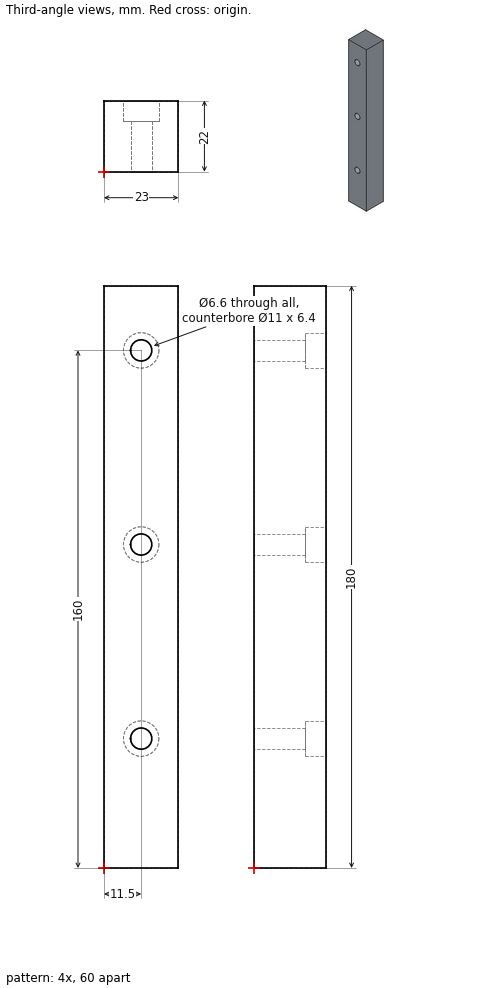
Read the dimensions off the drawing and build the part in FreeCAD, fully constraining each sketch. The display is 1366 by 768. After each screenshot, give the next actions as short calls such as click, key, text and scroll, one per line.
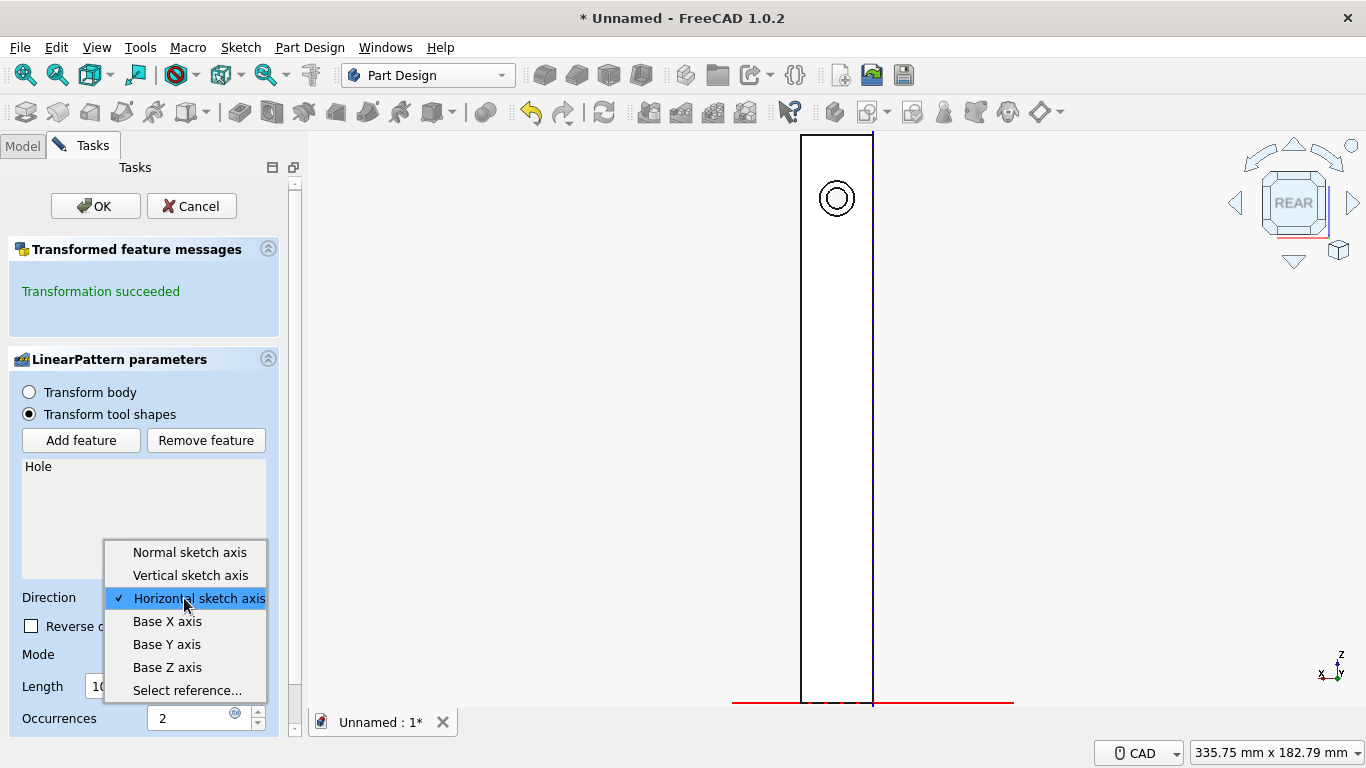
click(184, 668)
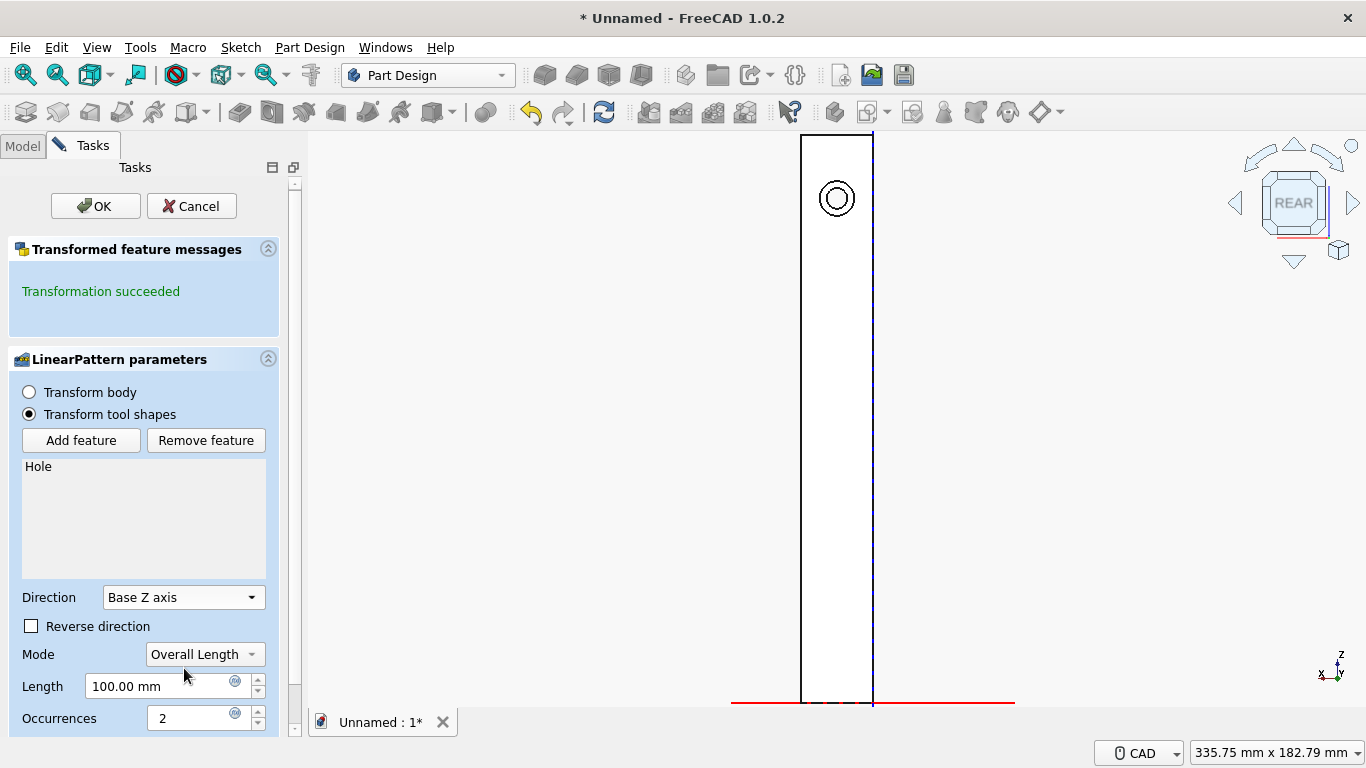
click(206, 654)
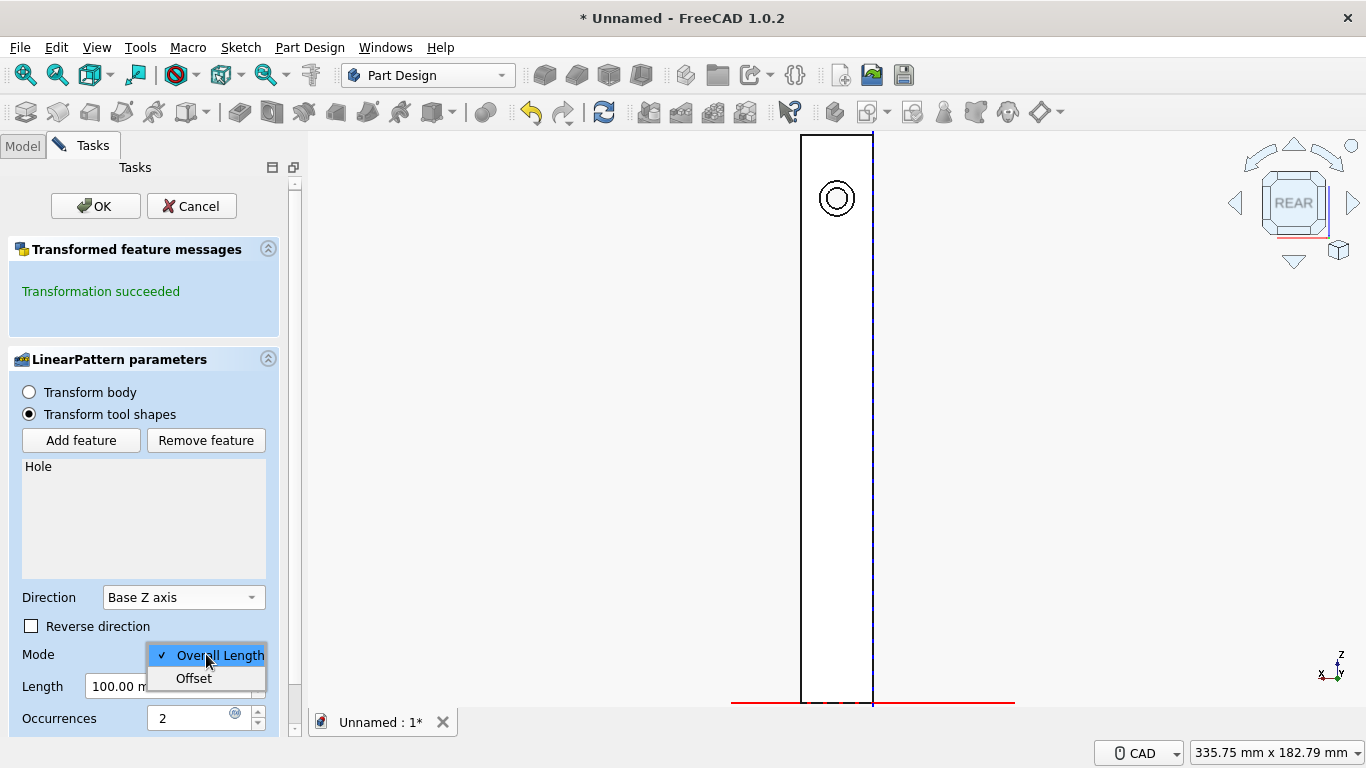
click(206, 678)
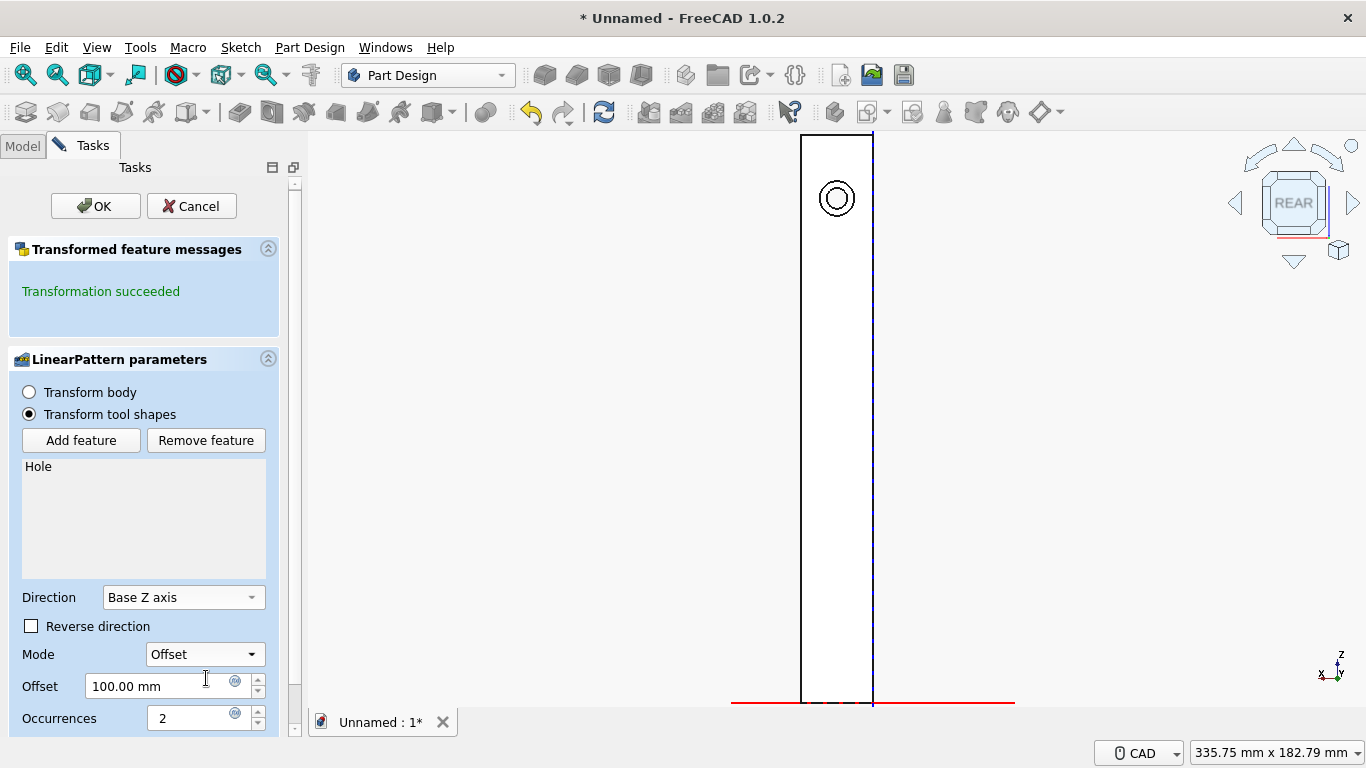
triple_click(168, 686)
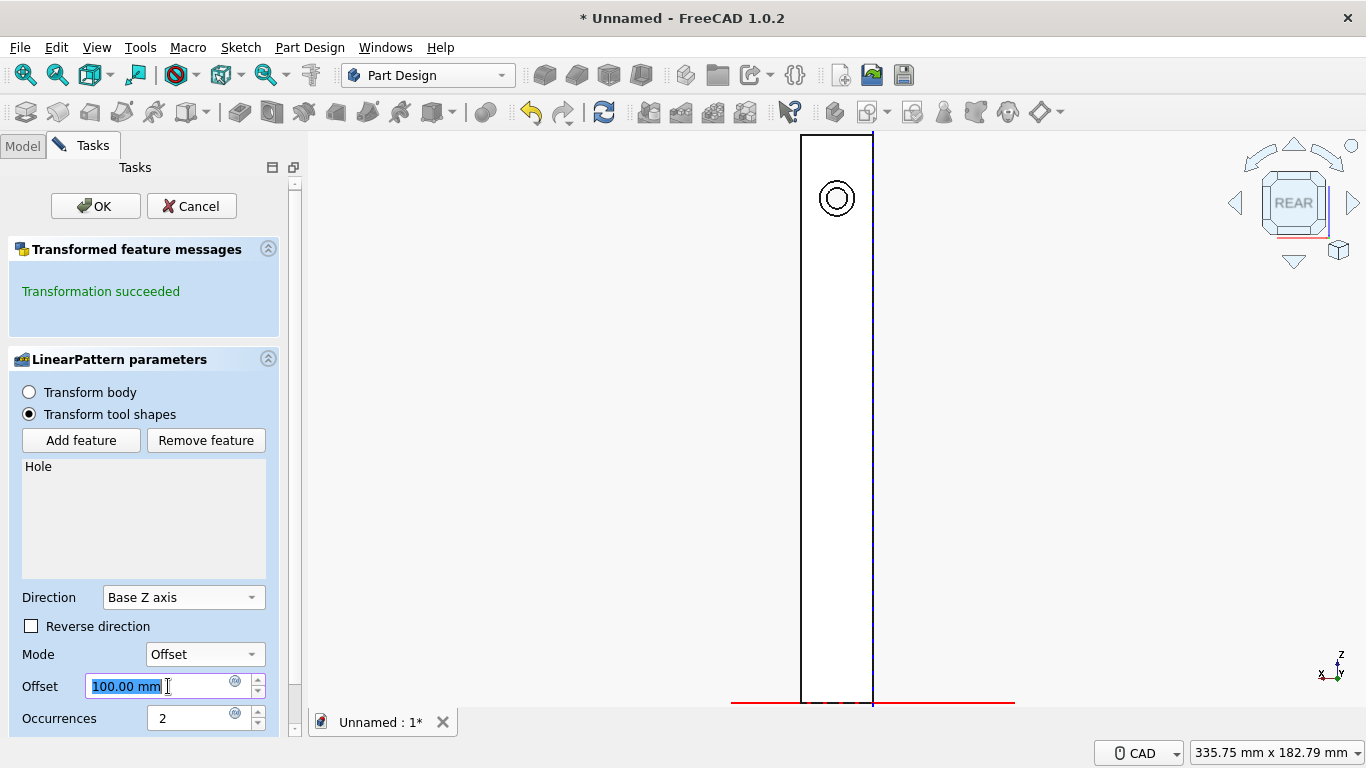
text(60)
key(Tab)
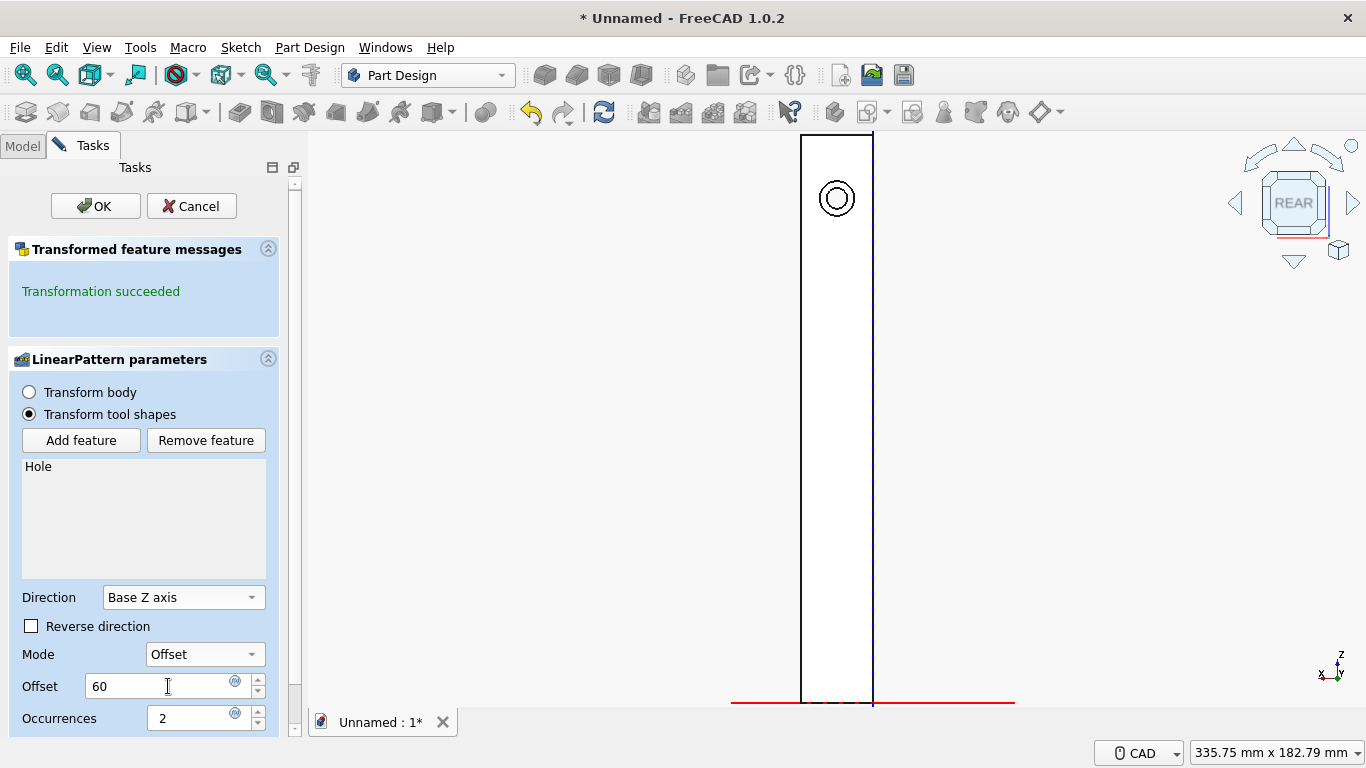
triple_click(198, 718)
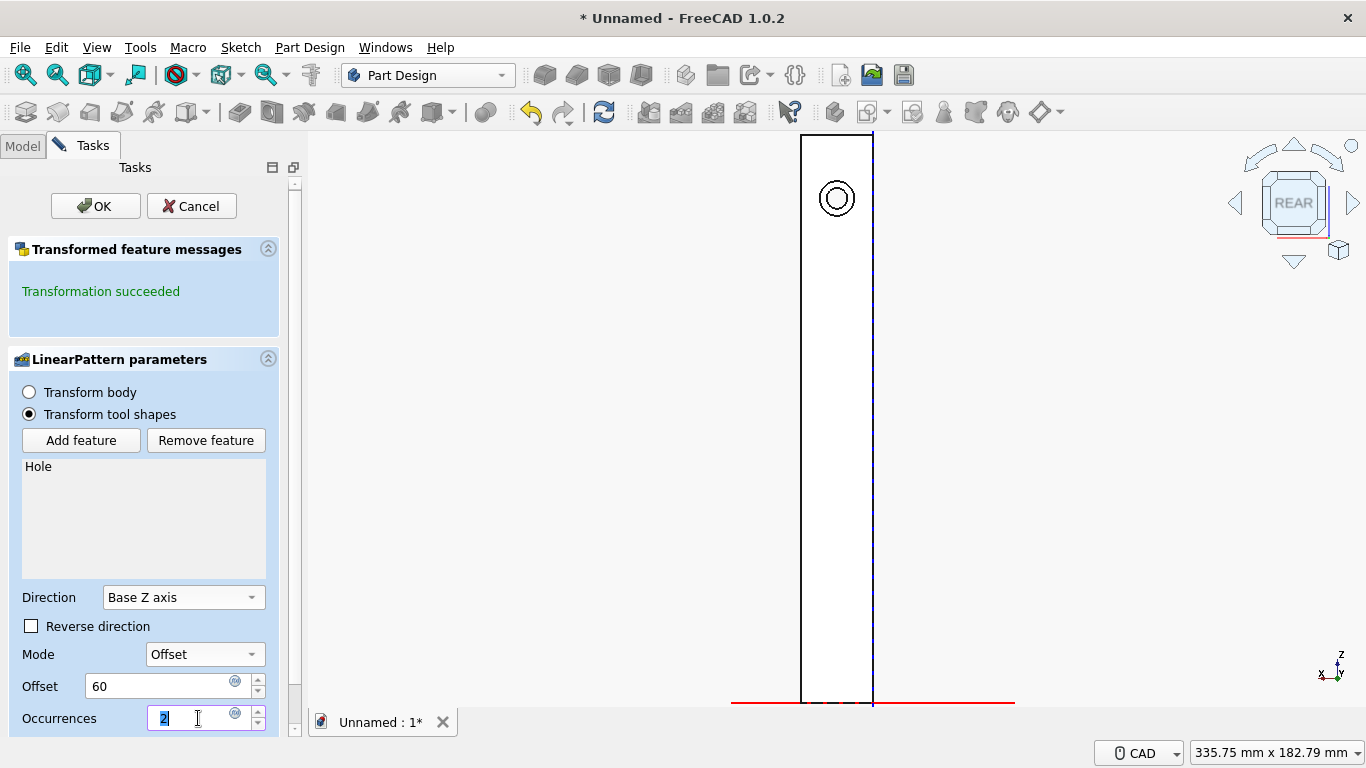
text(4)
key(Tab)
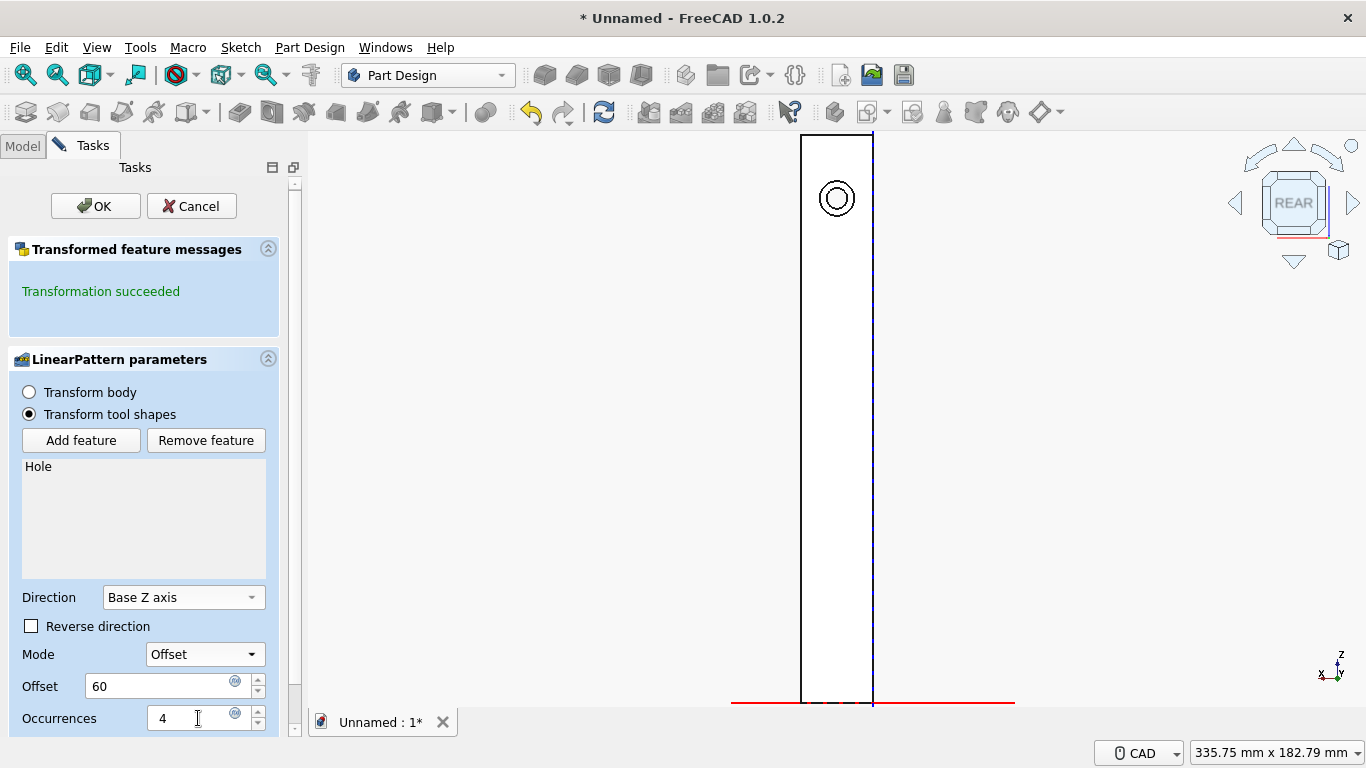
click(30, 626)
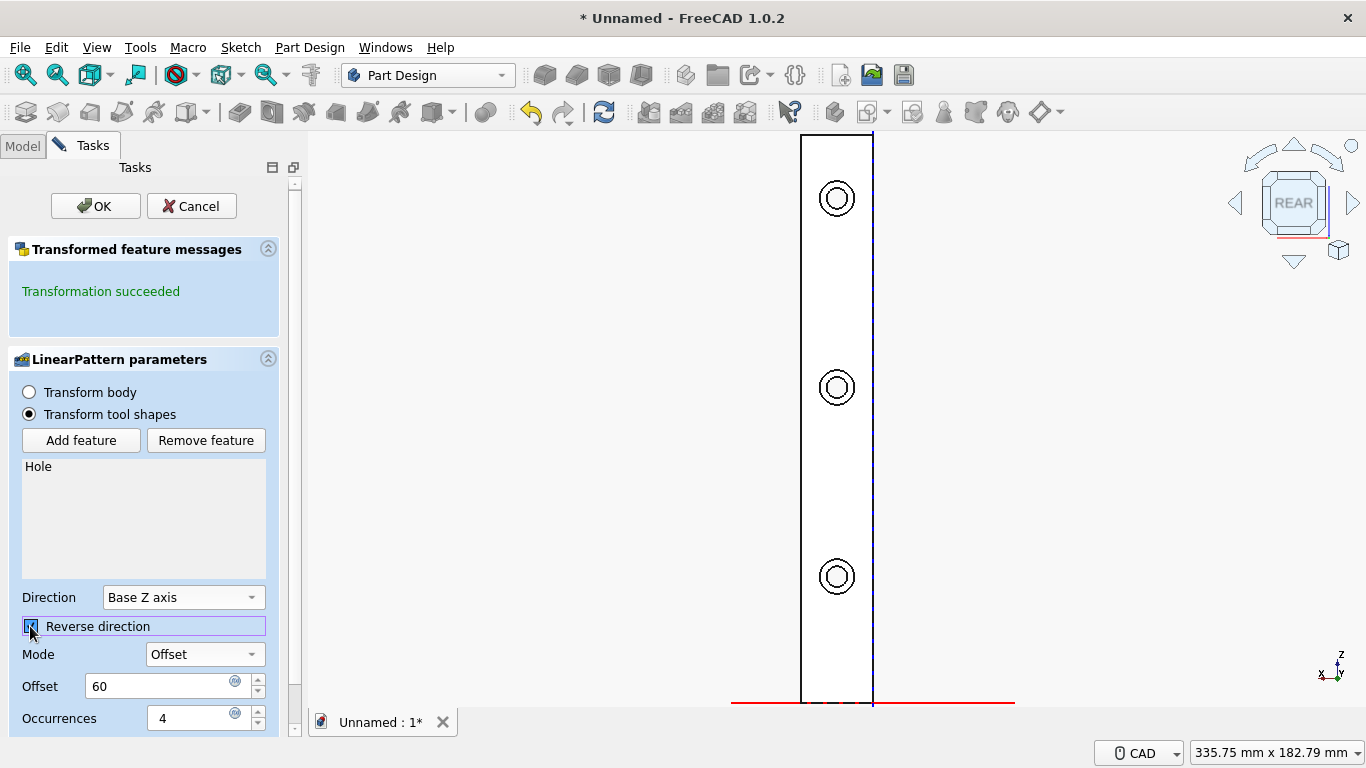
click(96, 206)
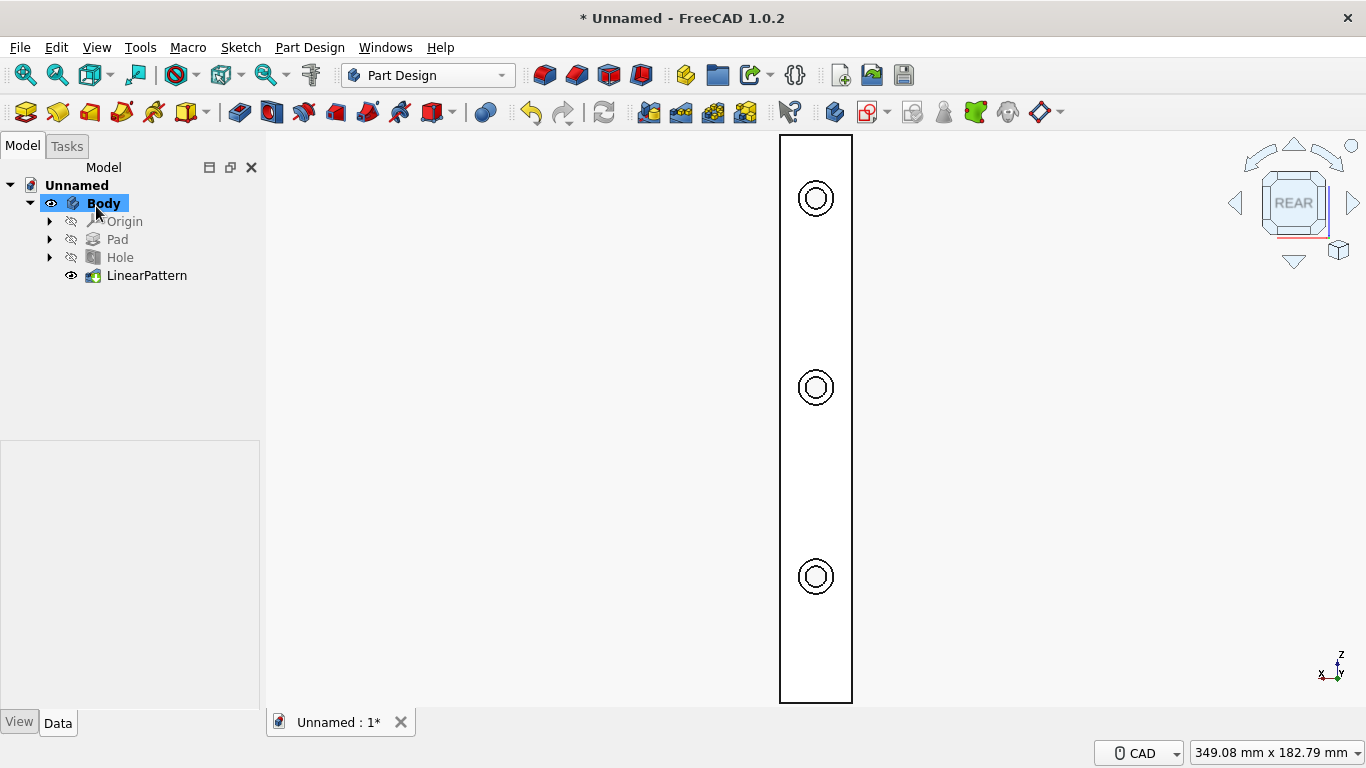
key(0)